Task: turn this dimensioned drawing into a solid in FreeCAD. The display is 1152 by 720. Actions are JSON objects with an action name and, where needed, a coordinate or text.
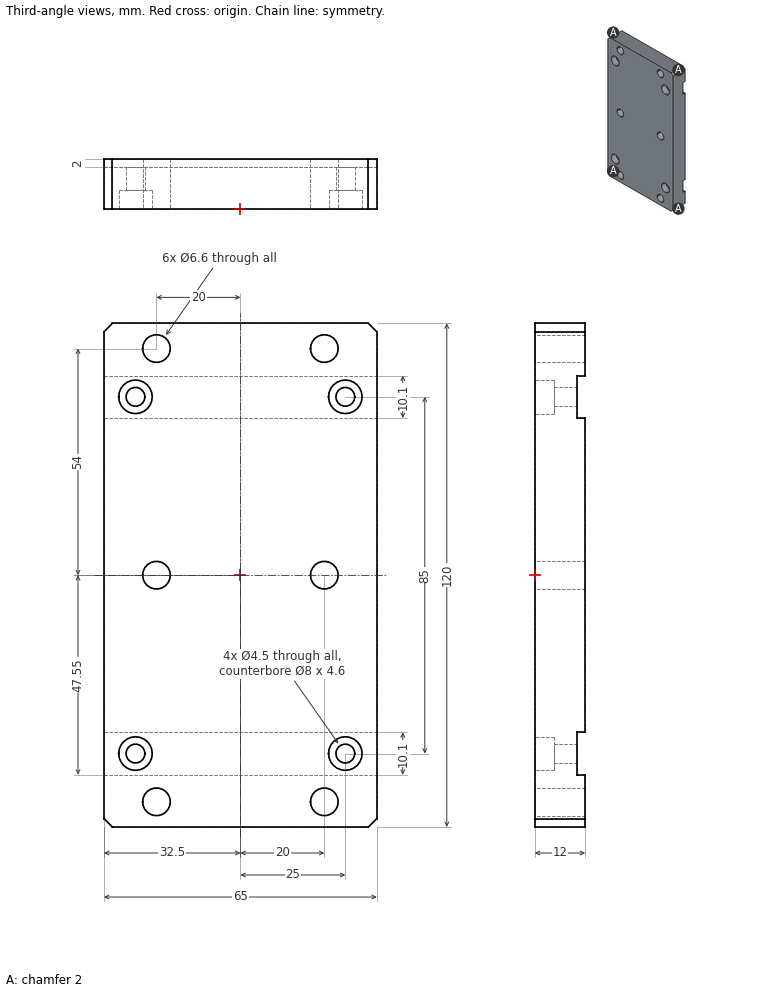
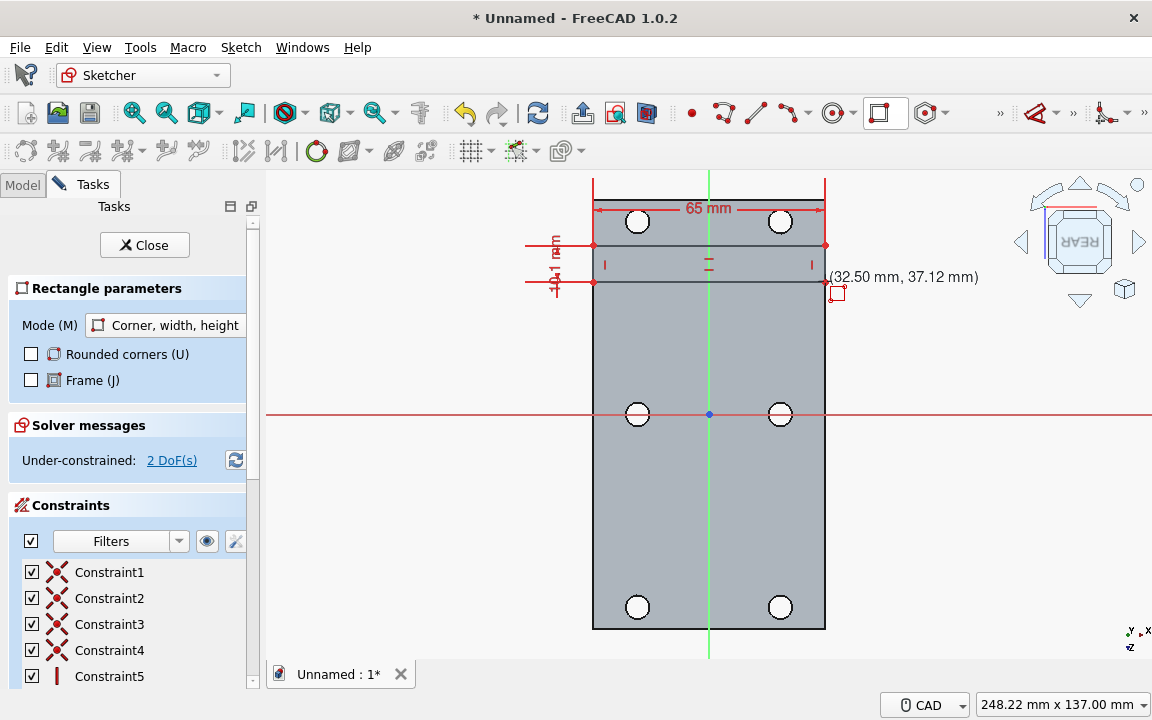
{"action": "left_click", "coordinate": [593, 548]}
{"action": "mouse_move", "coordinate": [825, 584]}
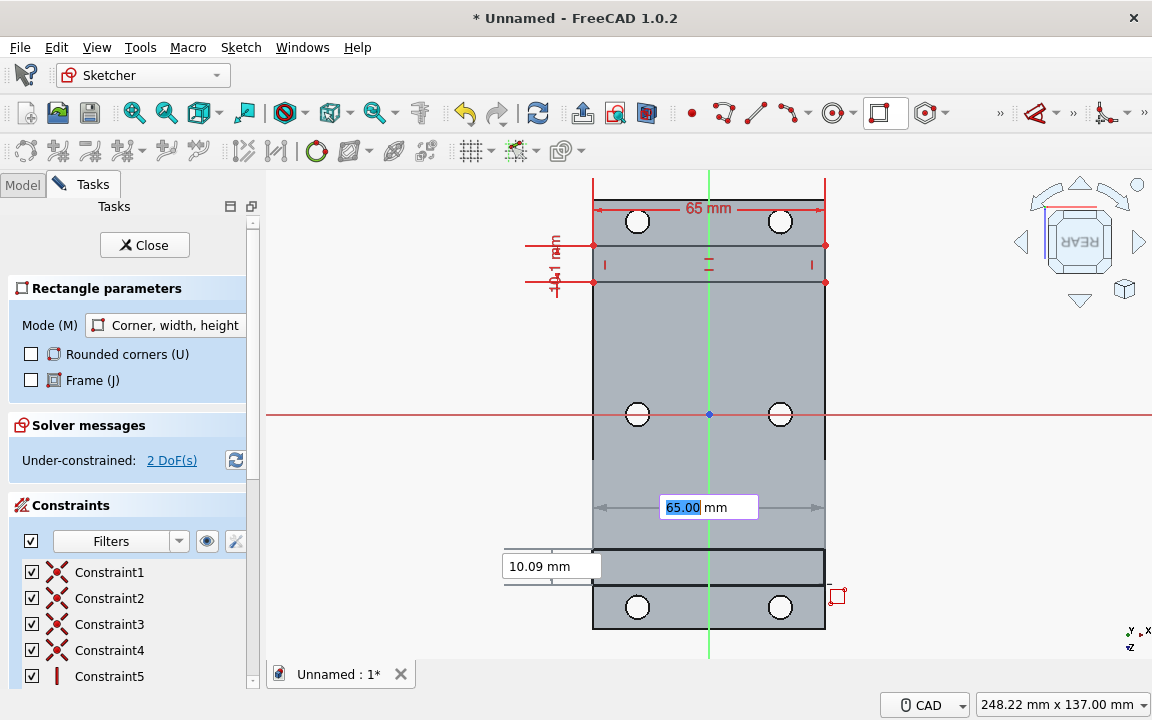
{"action": "type", "text": "65"}
{"action": "key", "text": "Tab"}
{"action": "type", "text": "10.1"}
{"action": "key", "text": "Return"}
{"action": "key", "text": "Escape"}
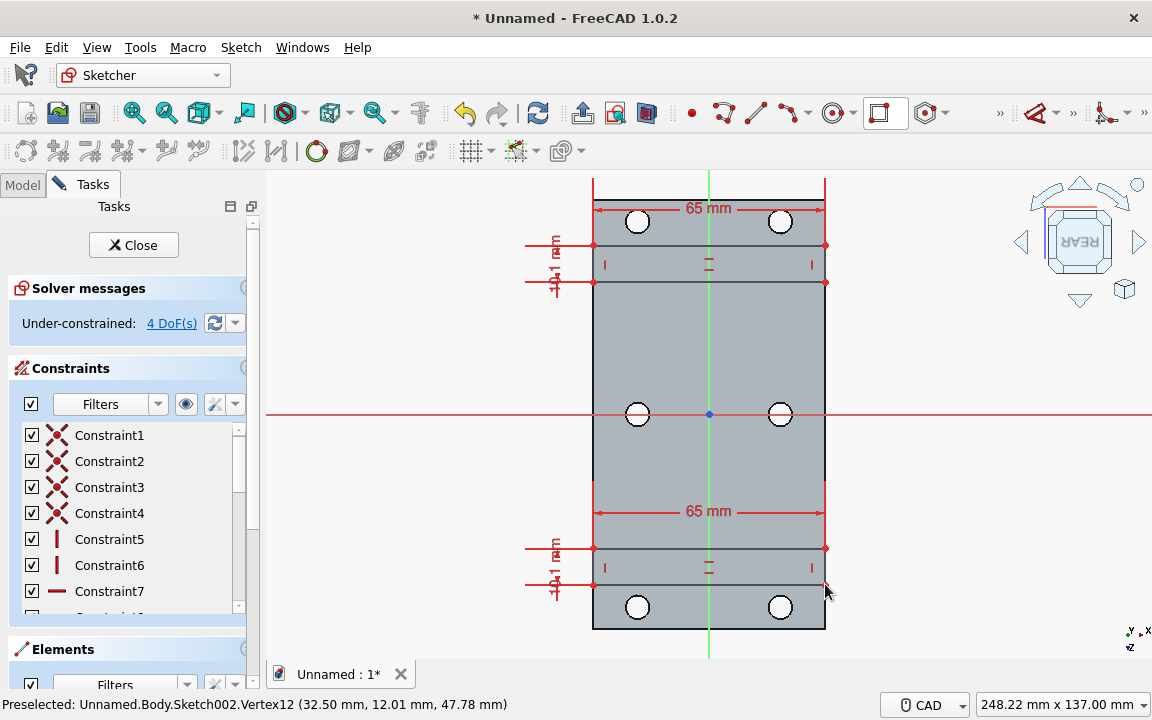
{"action": "left_click", "coordinate": [593, 282]}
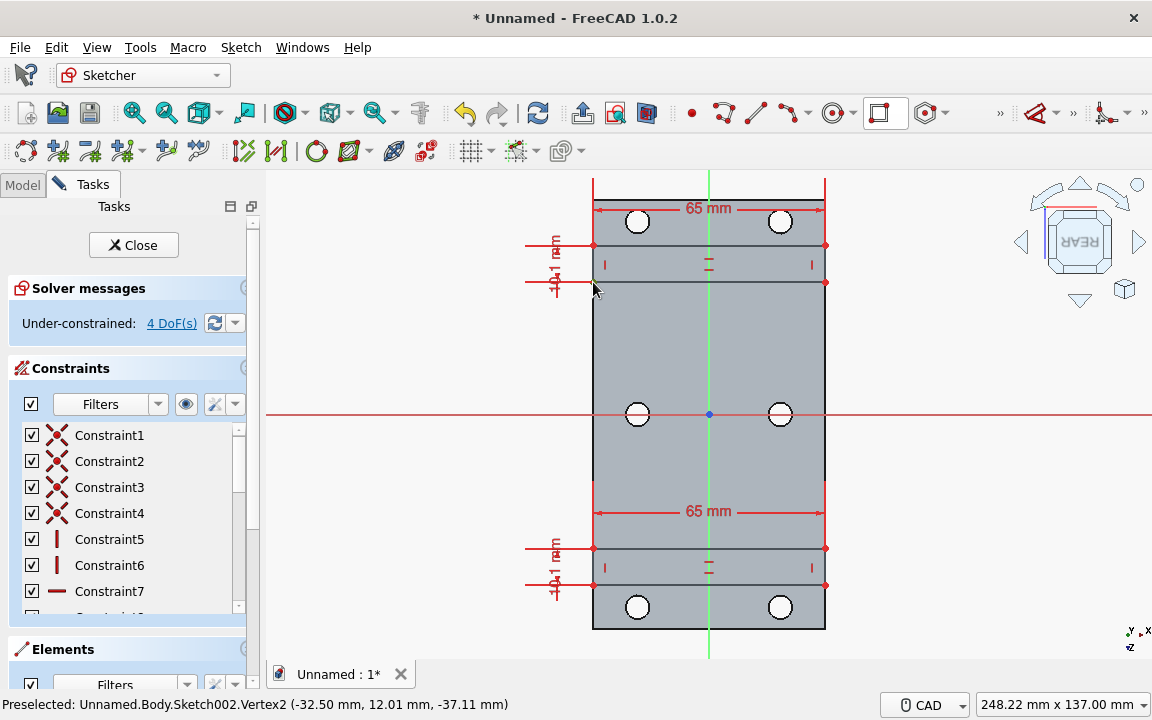
{"action": "left_click", "coordinate": [593, 549]}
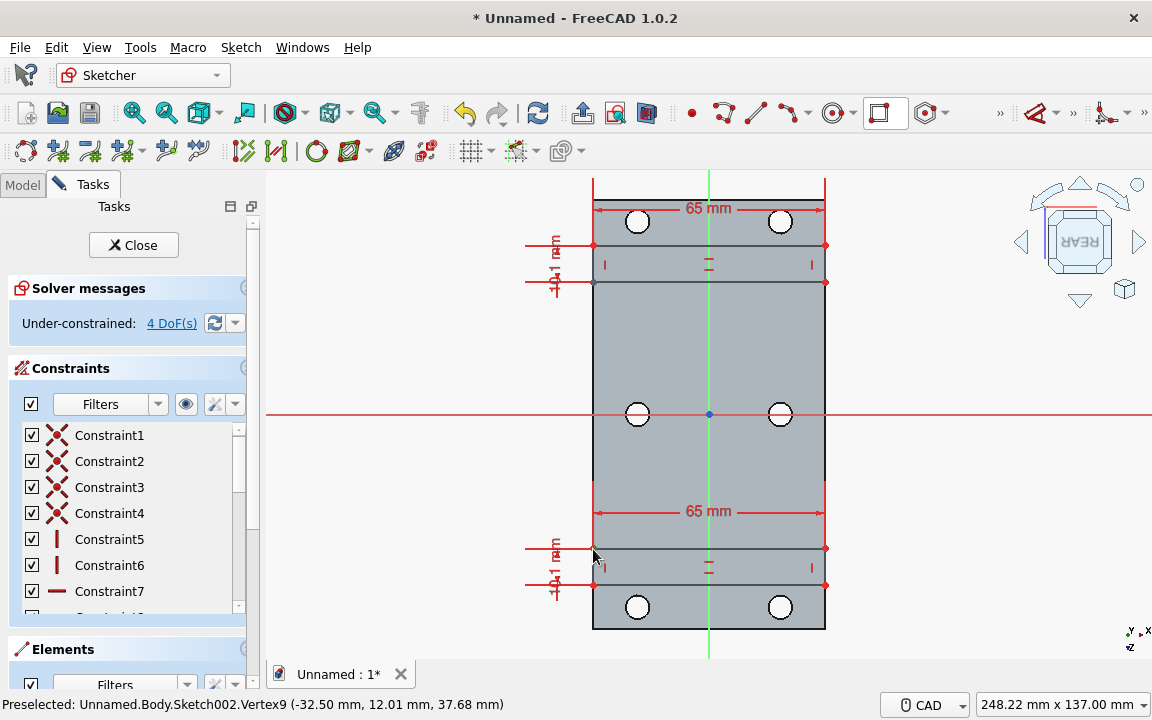
{"action": "left_click", "coordinate": [344, 414]}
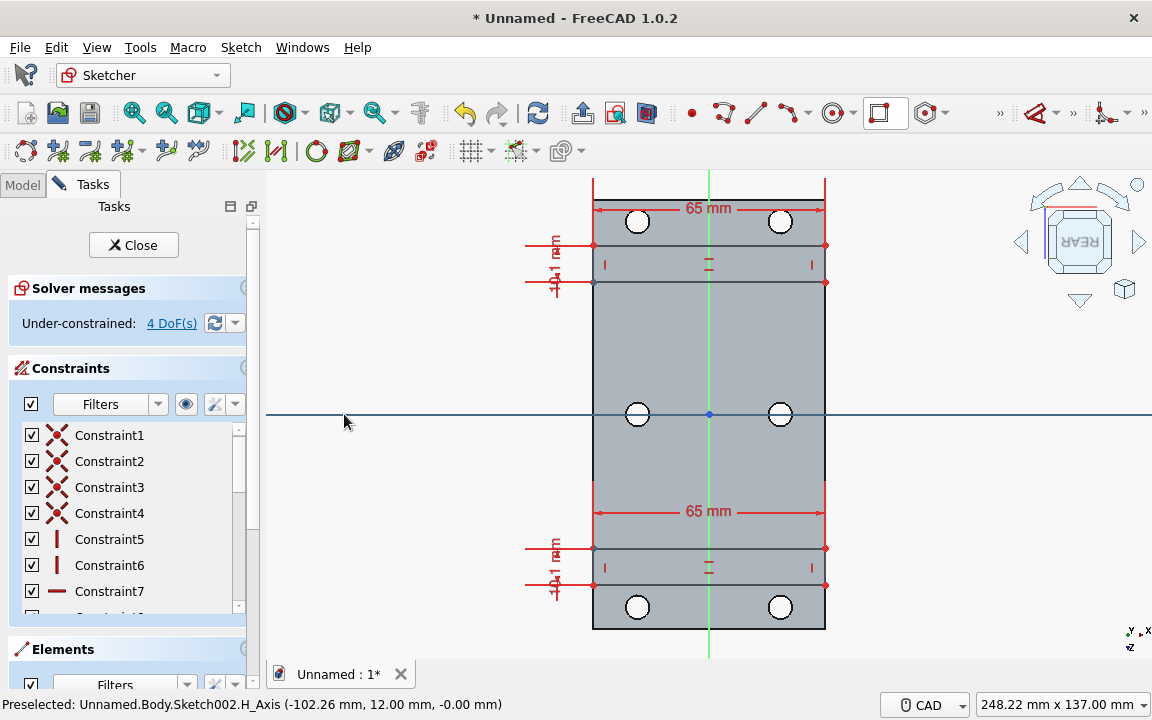
{"action": "key", "text": "s"}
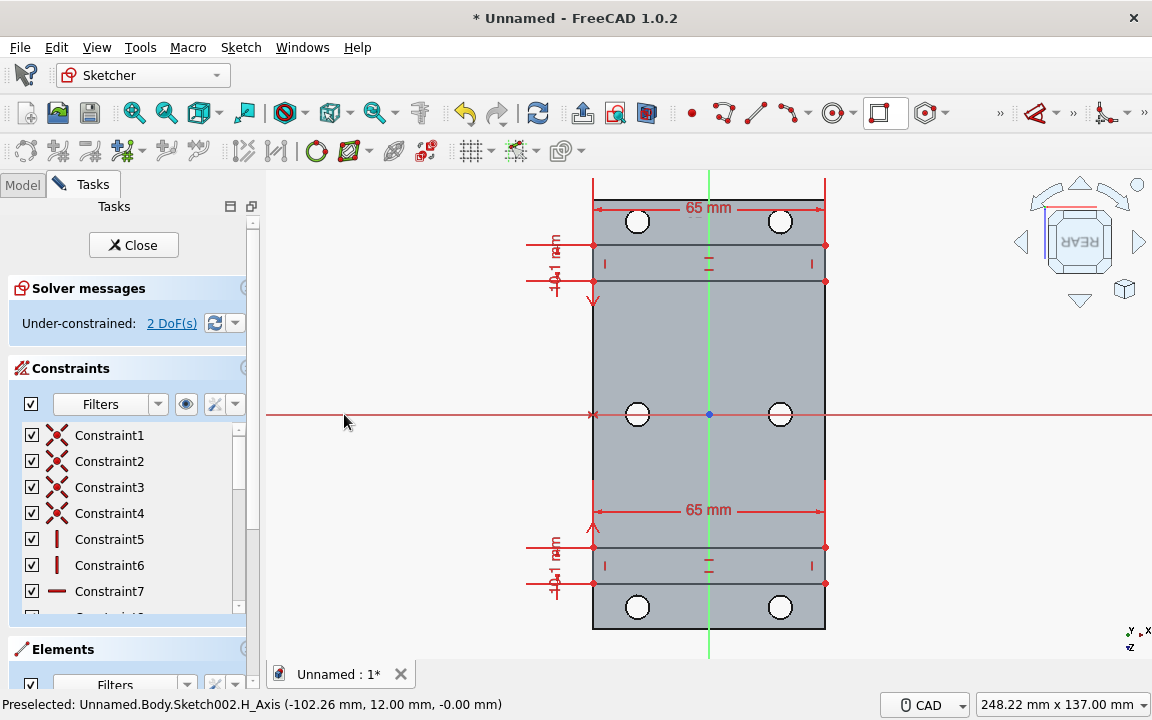
{"action": "key", "text": "d"}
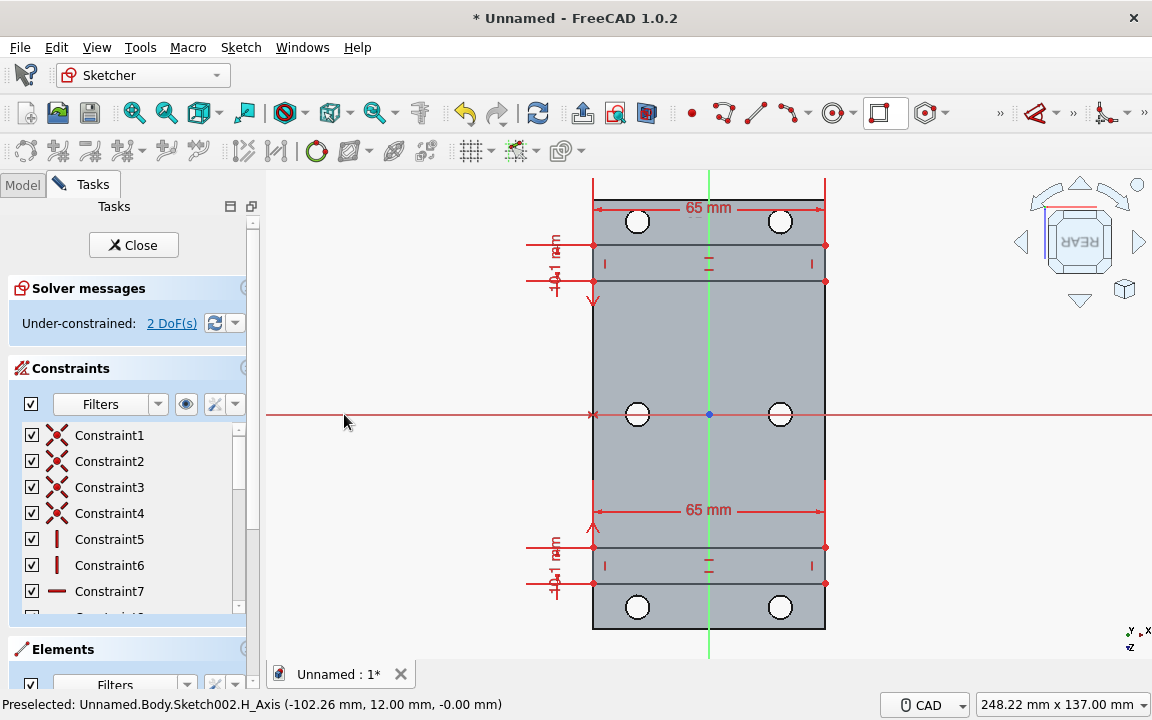
{"action": "left_click", "coordinate": [593, 245]}
{"action": "left_click", "coordinate": [651, 211]}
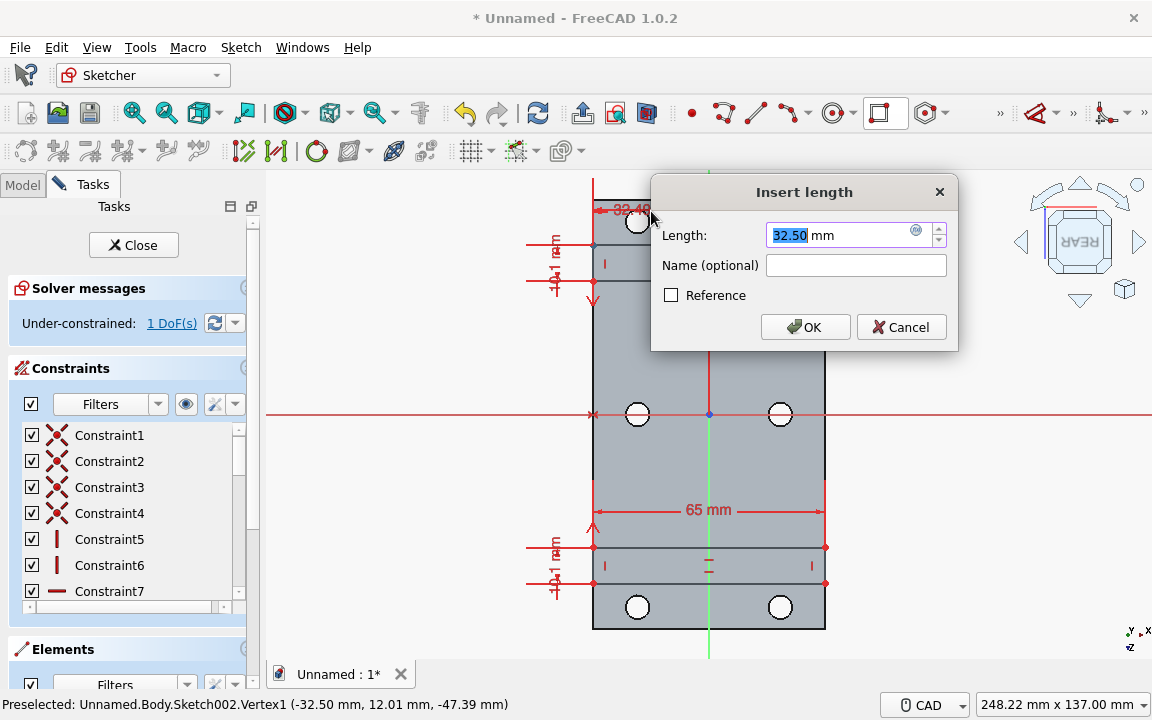
{"action": "type", "text": "32.5"}
{"action": "key", "text": "Return"}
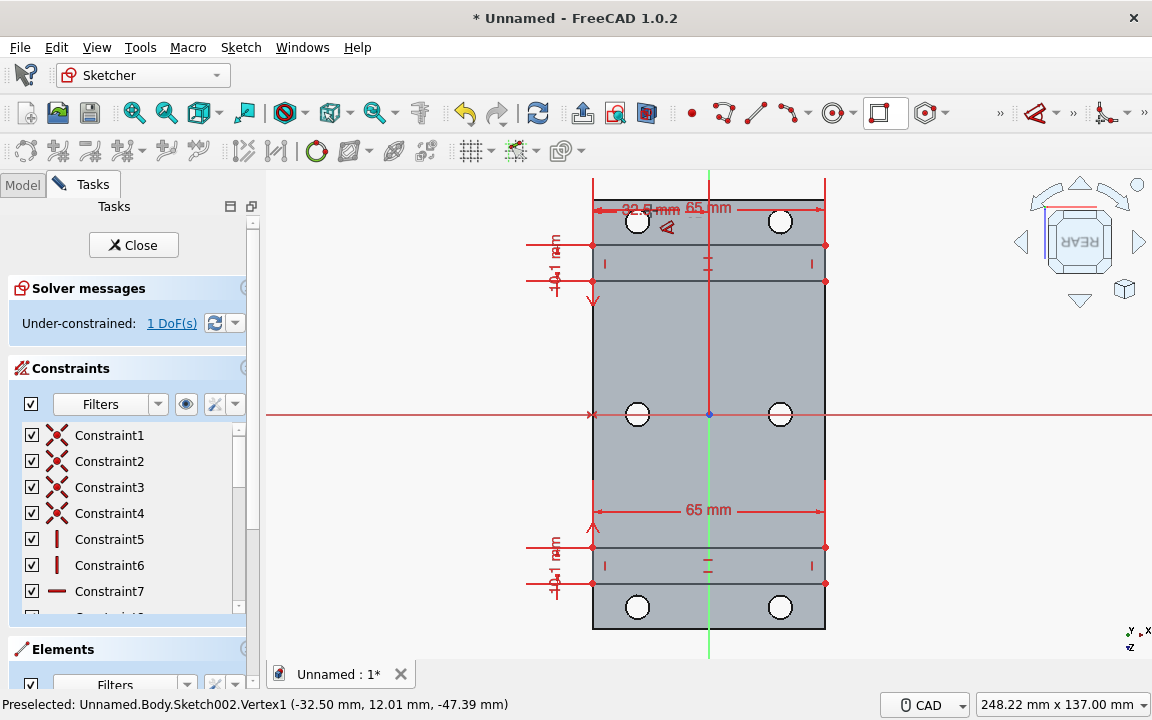
{"action": "left_click", "coordinate": [593, 245]}
{"action": "left_click", "coordinate": [559, 330]}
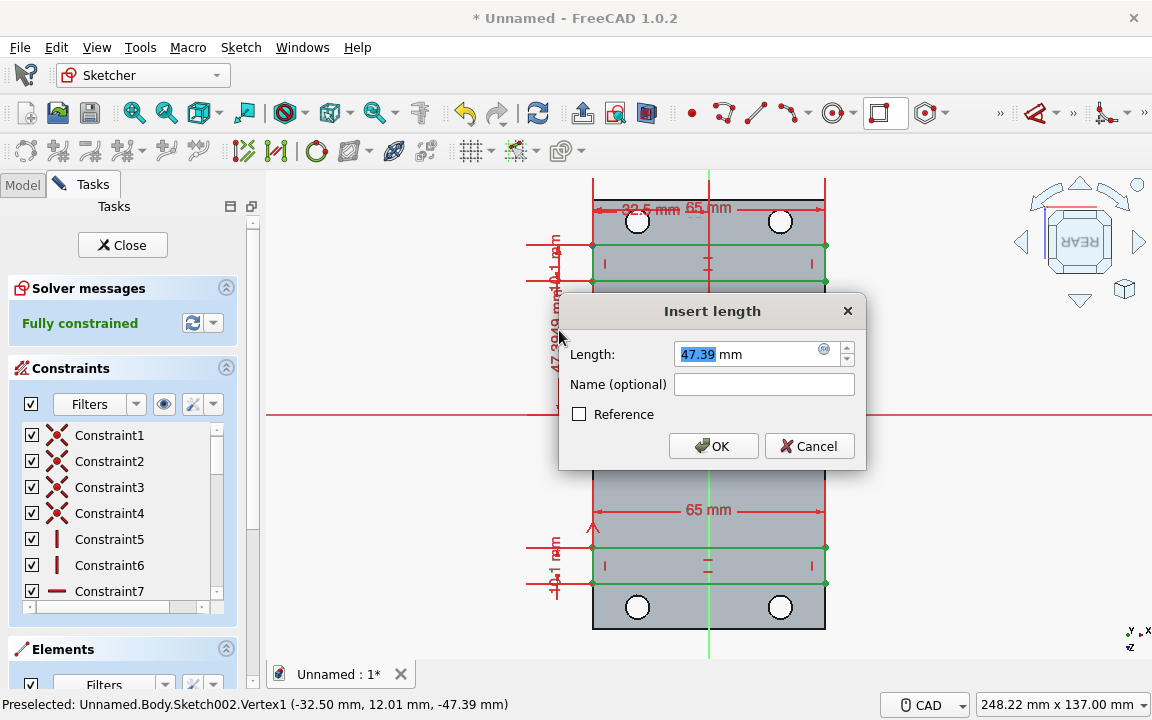
{"action": "type", "text": "47.55"}
{"action": "key", "text": "Return"}
{"action": "key", "text": "Escape"}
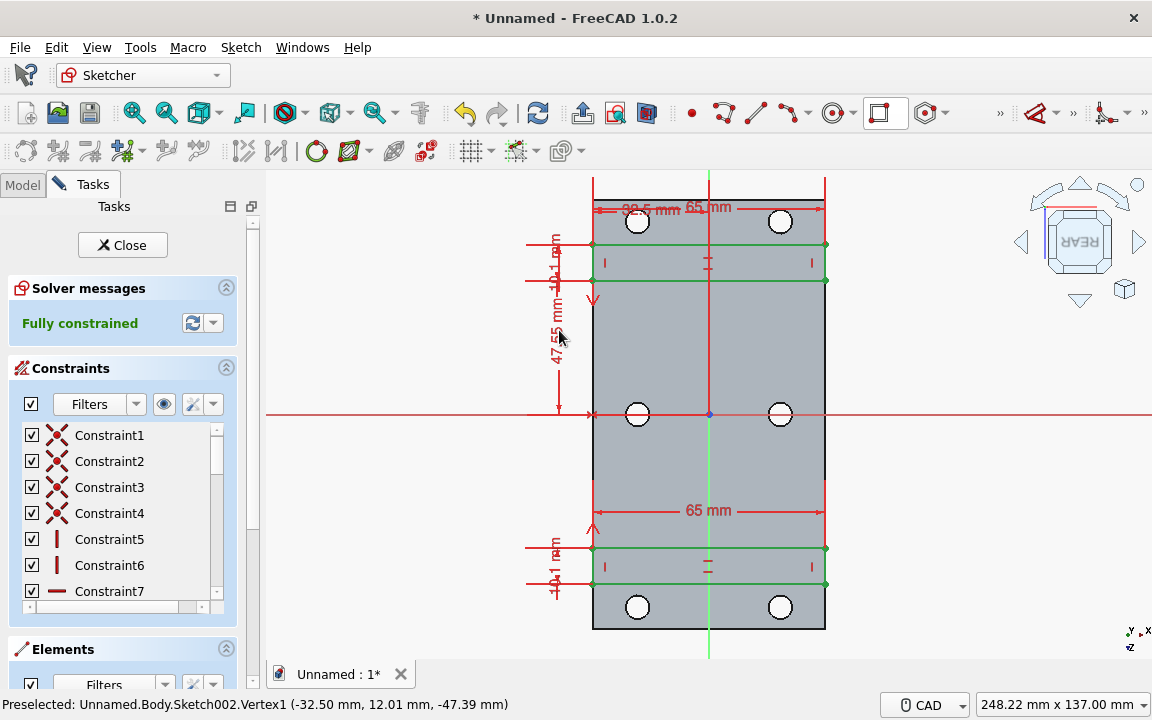
{"action": "left_click", "coordinate": [123, 245]}